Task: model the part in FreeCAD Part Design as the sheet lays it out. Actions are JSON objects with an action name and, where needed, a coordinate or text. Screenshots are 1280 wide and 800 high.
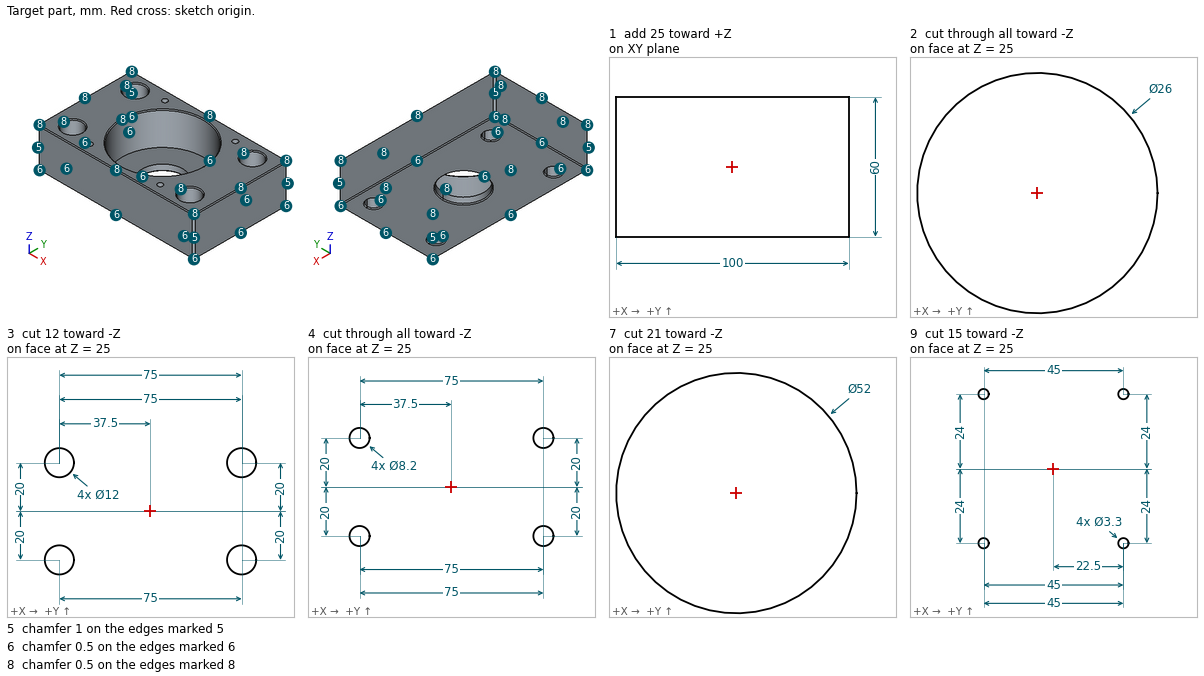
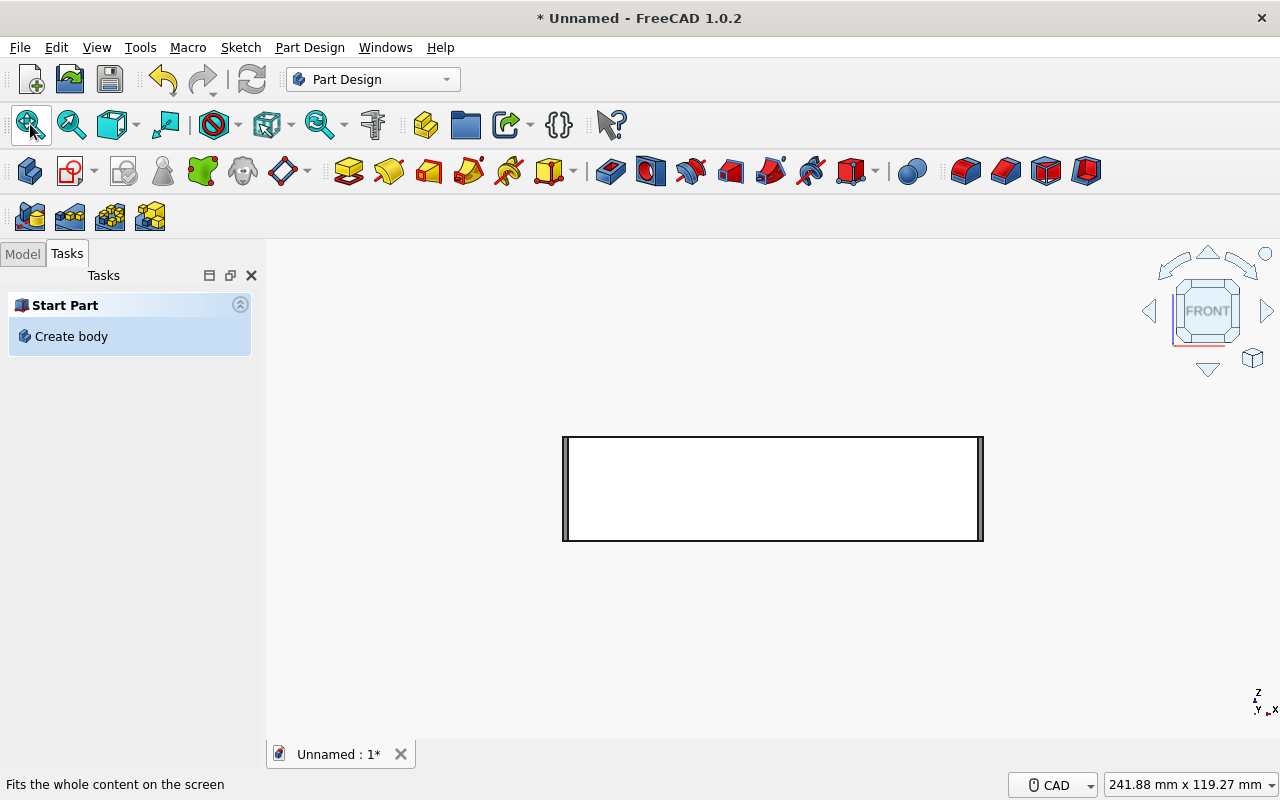
{"action": "key", "text": "3"}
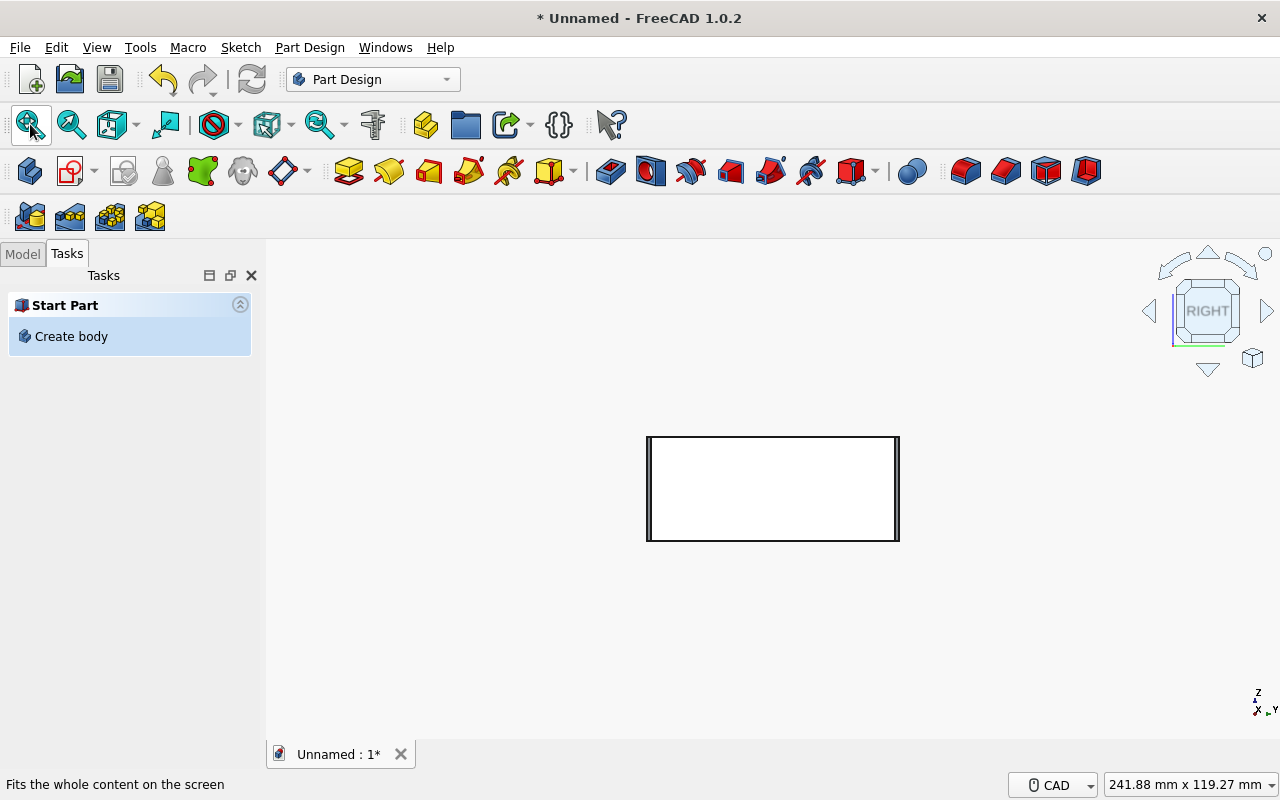
{"action": "key", "text": "v f"}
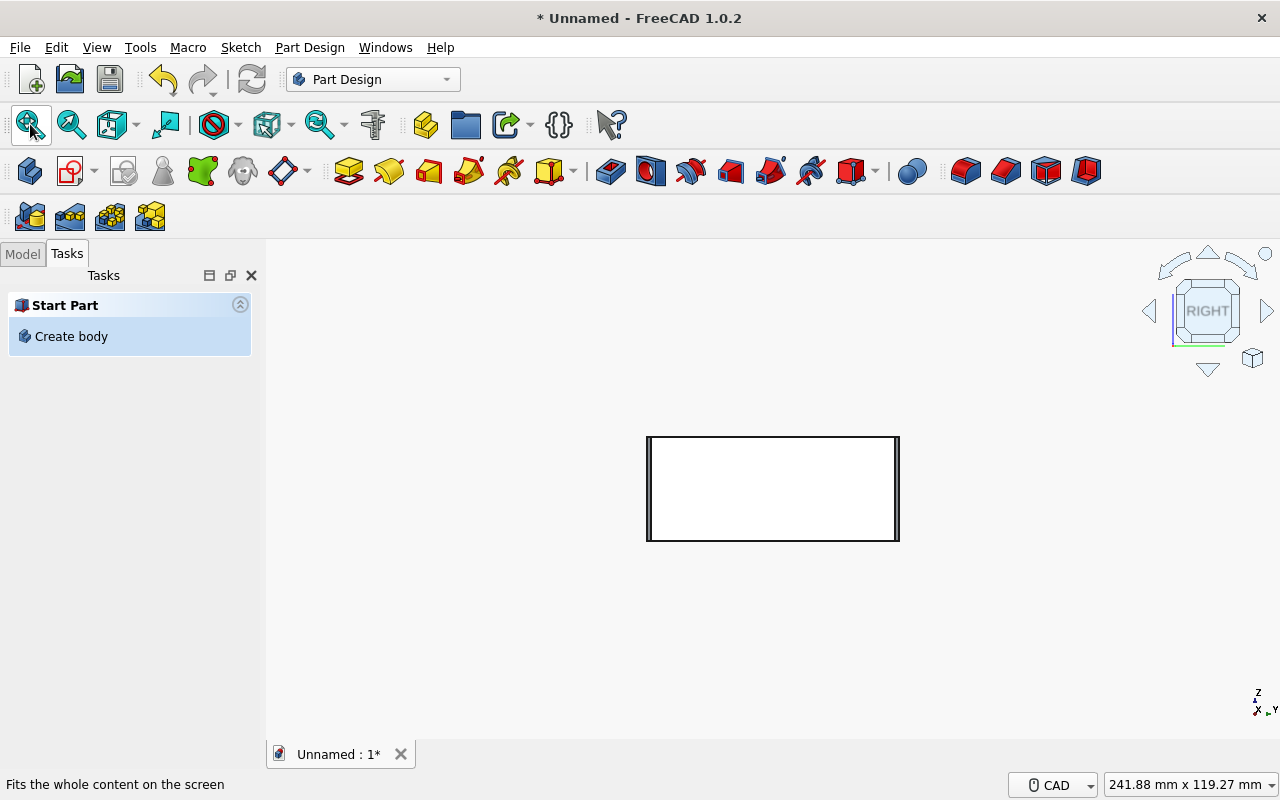
{"action": "key", "text": "5"}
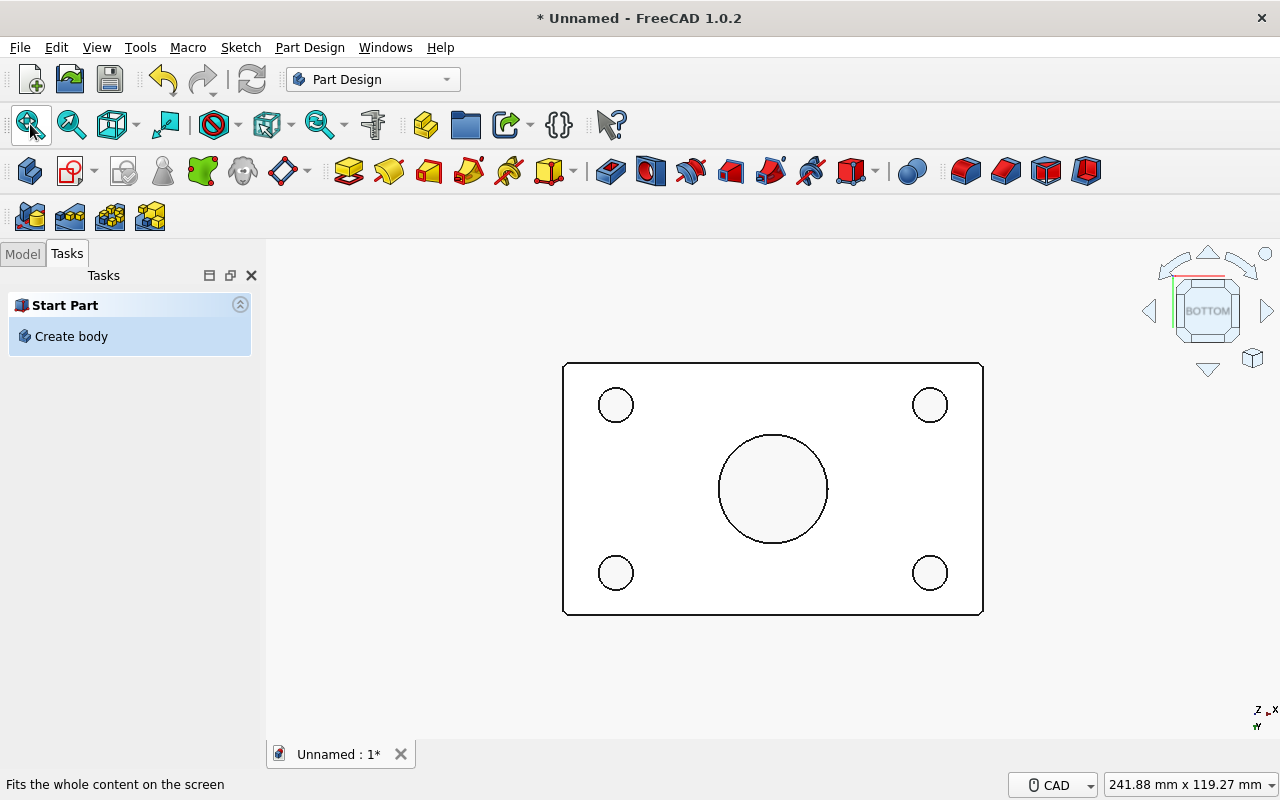
{"action": "left_click", "coordinate": [653, 488]}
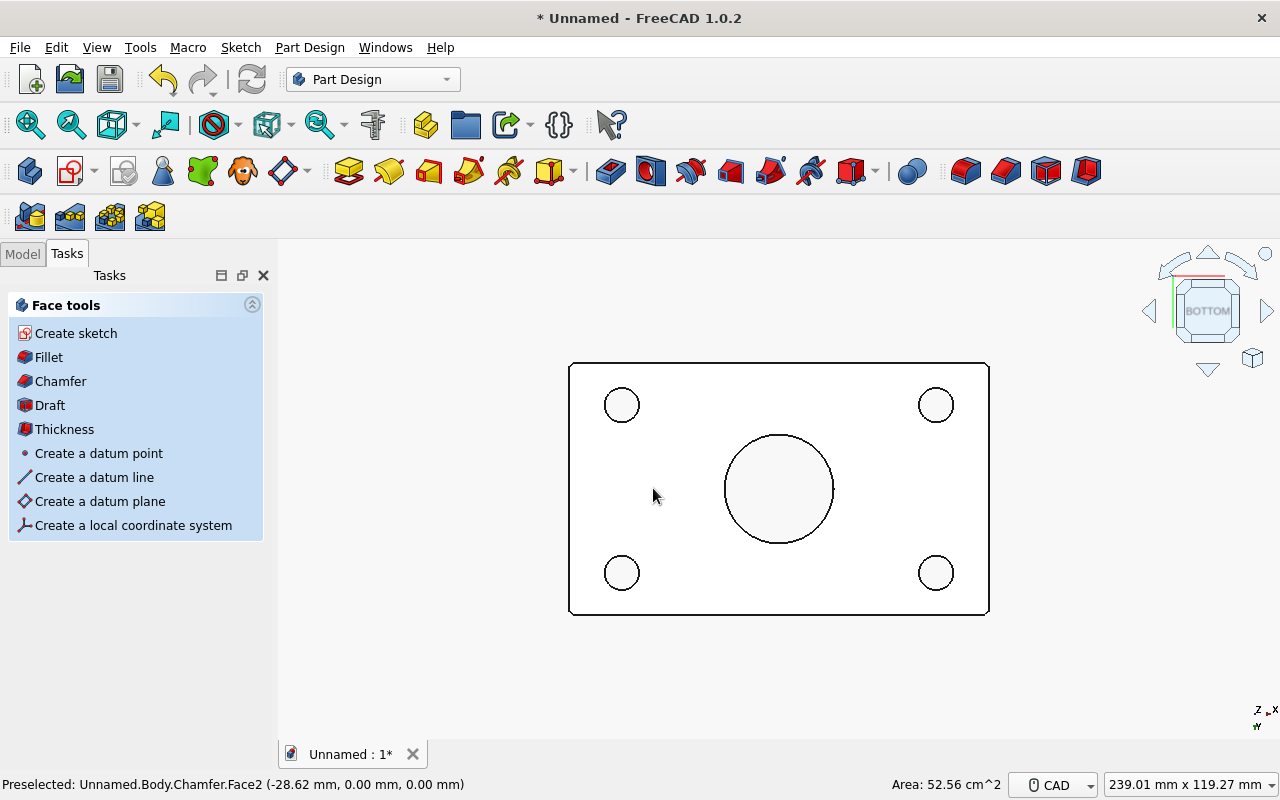
{"action": "left_click", "coordinate": [1006, 172]}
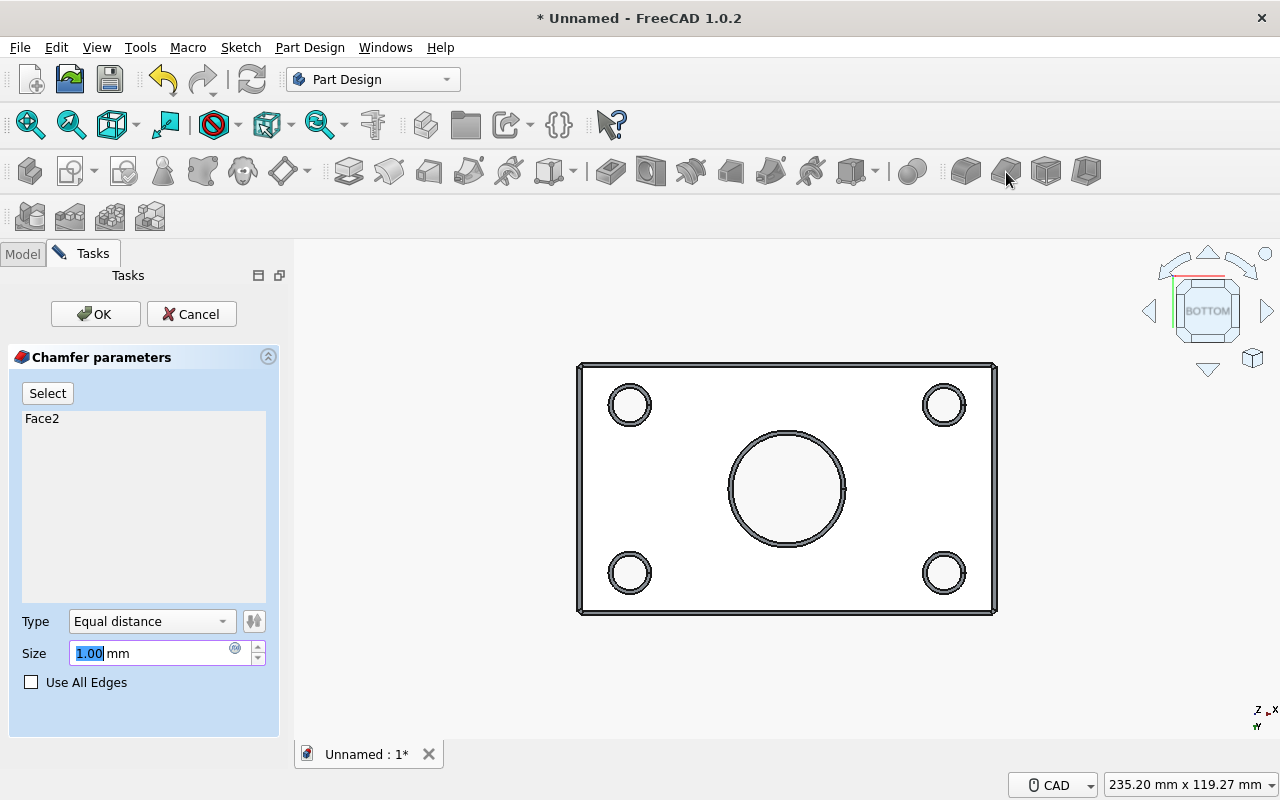
{"action": "type", "text": "0.5"}
{"action": "key", "text": "Tab"}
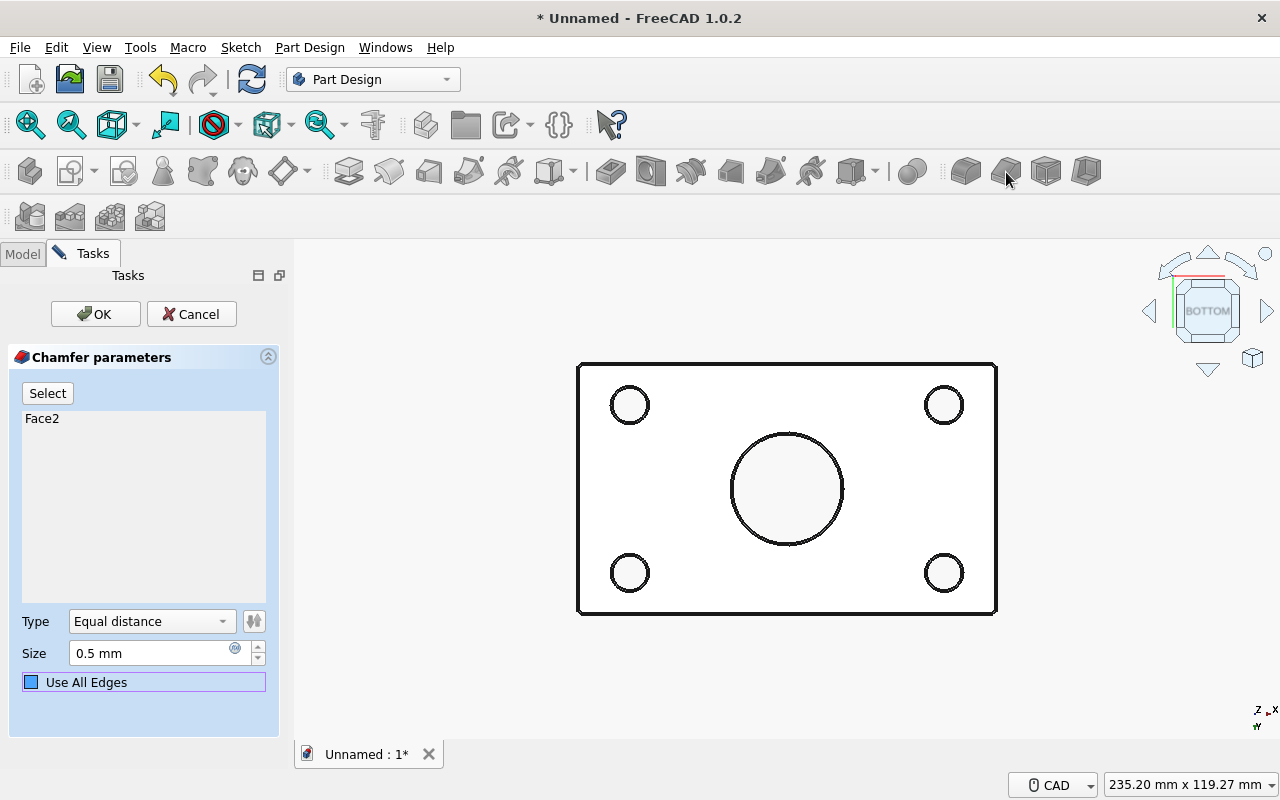
{"action": "left_click", "coordinate": [96, 314]}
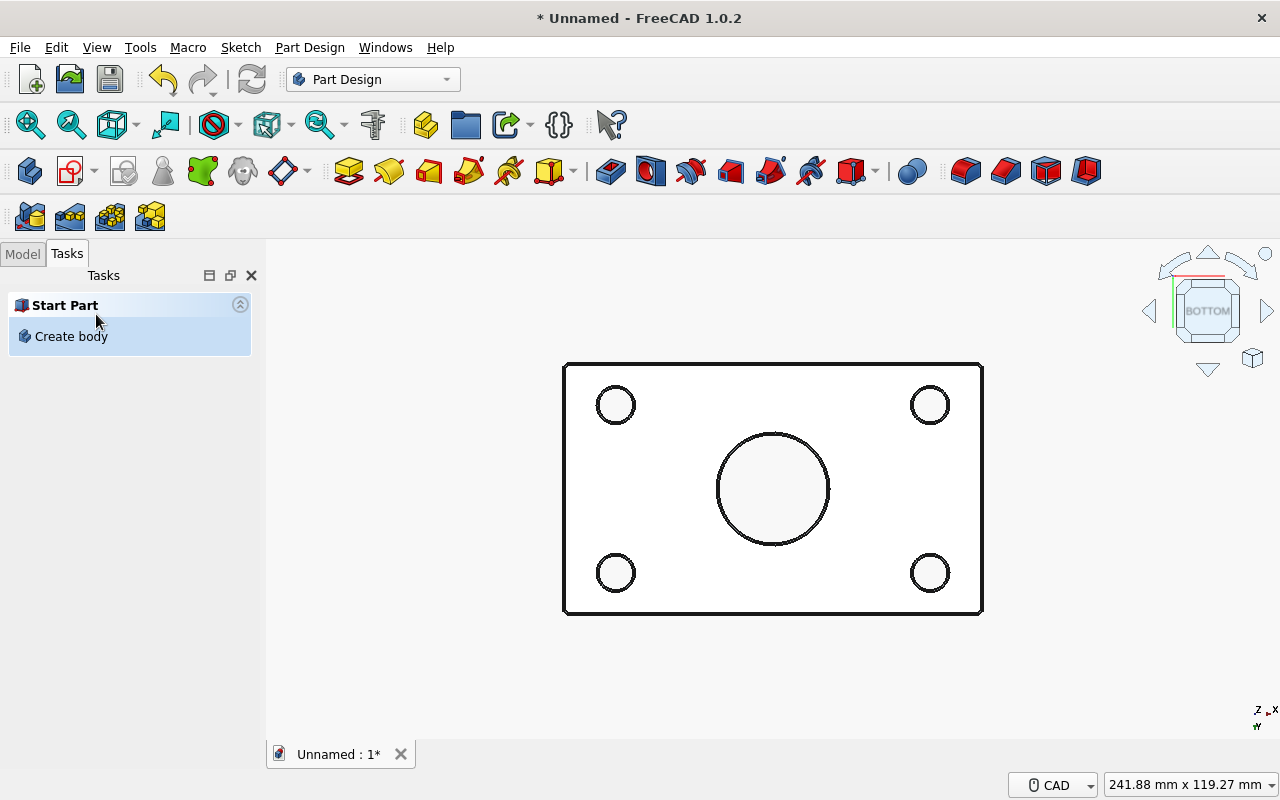
{"action": "key", "text": "0"}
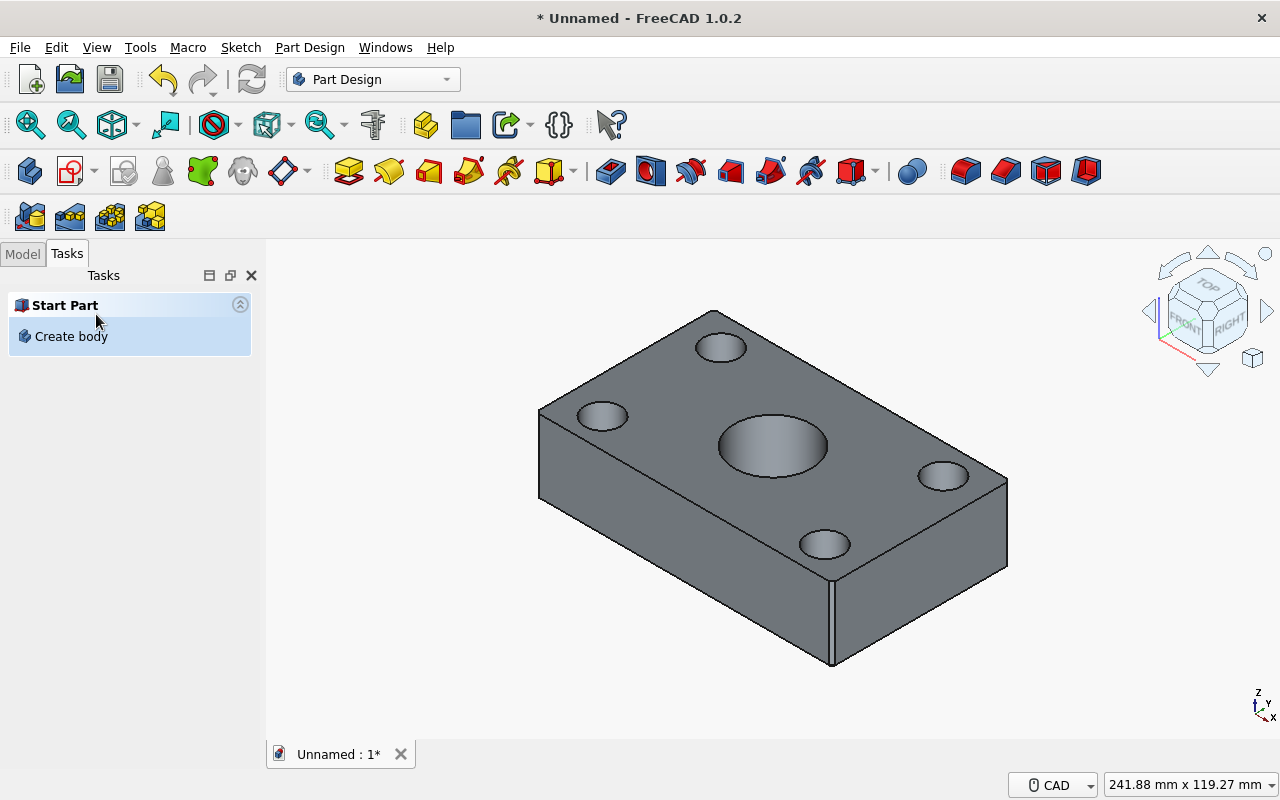
{"action": "left_click", "coordinate": [688, 396]}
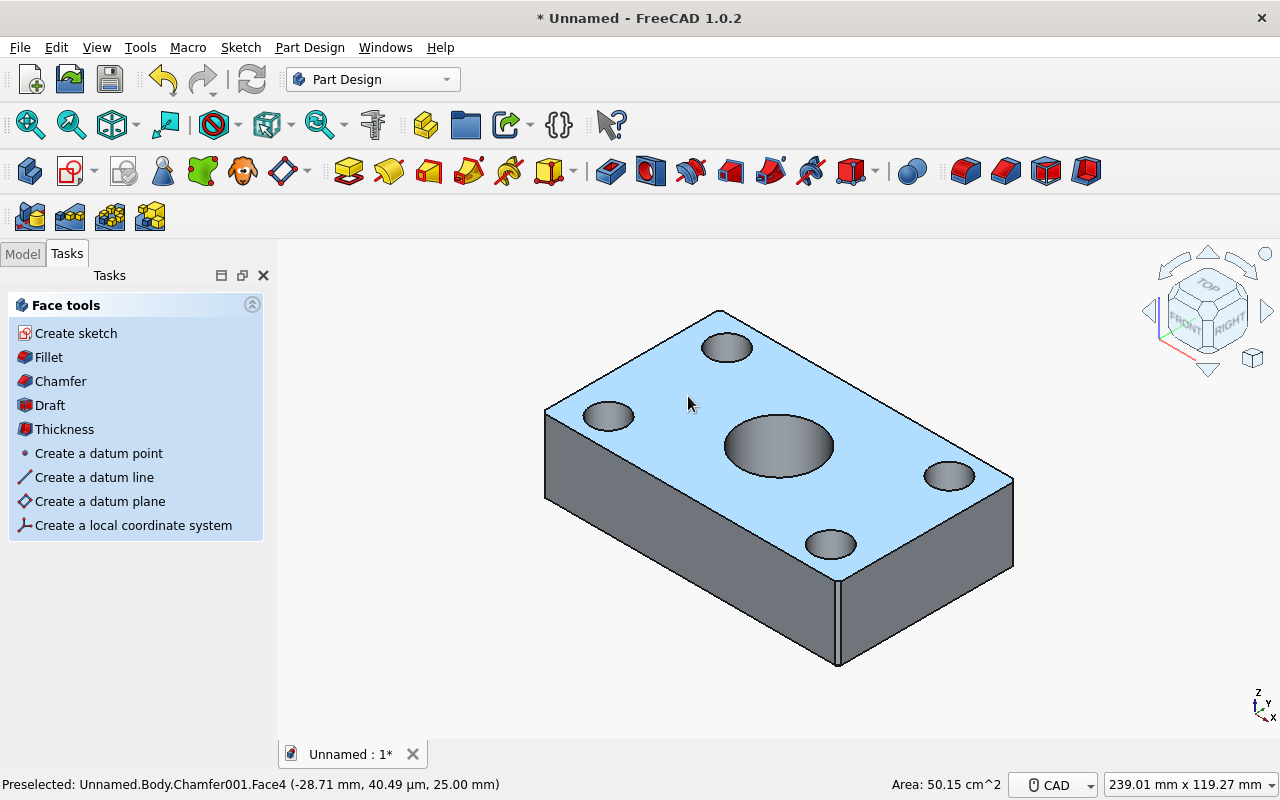
{"action": "left_click", "coordinate": [70, 172]}